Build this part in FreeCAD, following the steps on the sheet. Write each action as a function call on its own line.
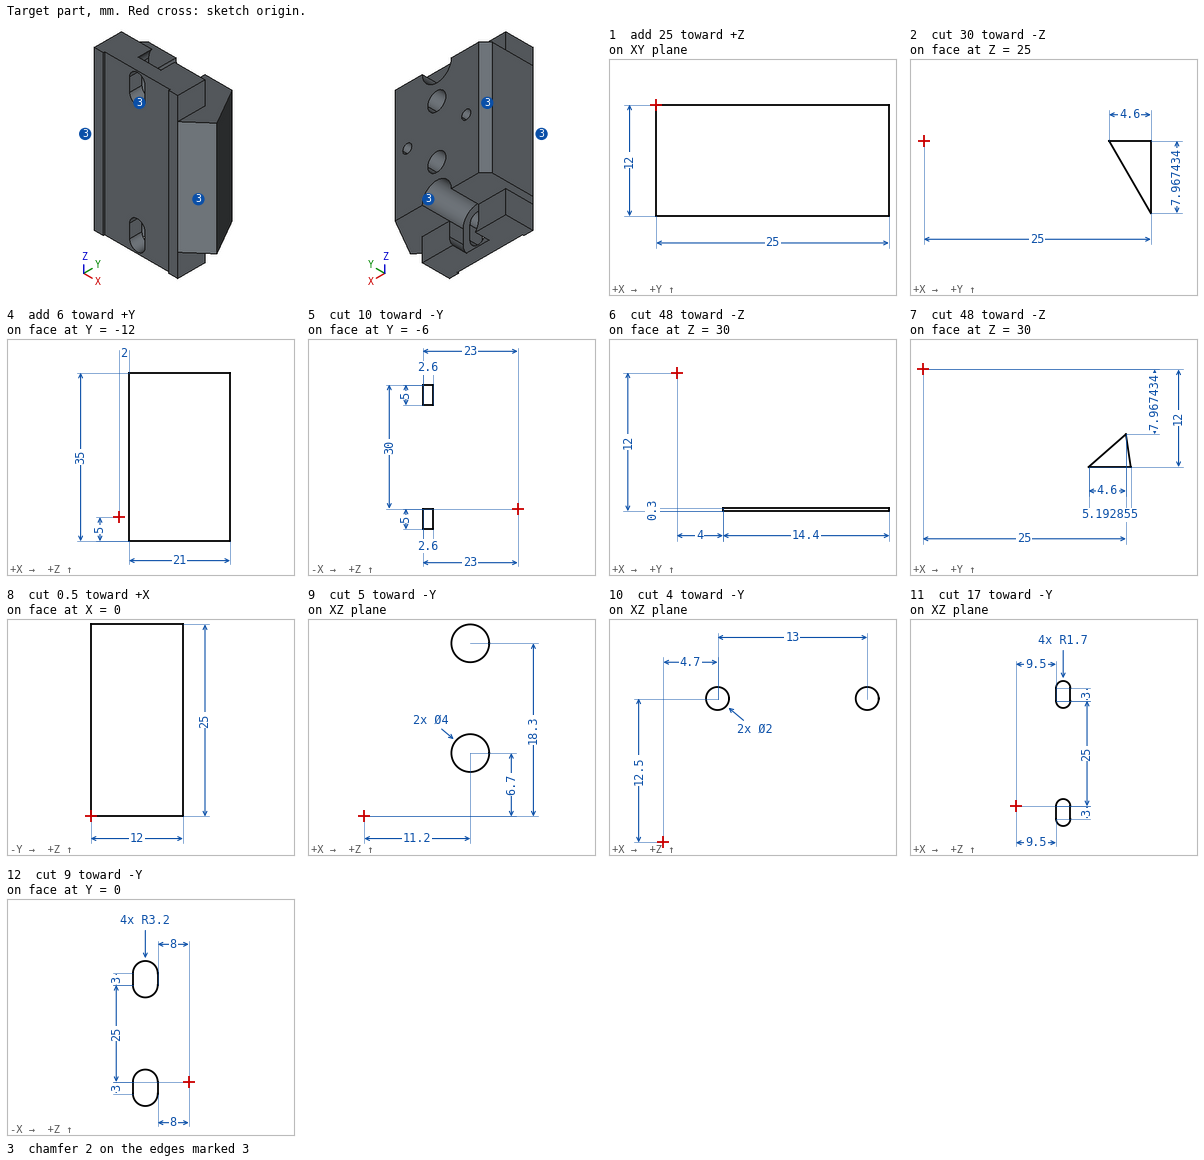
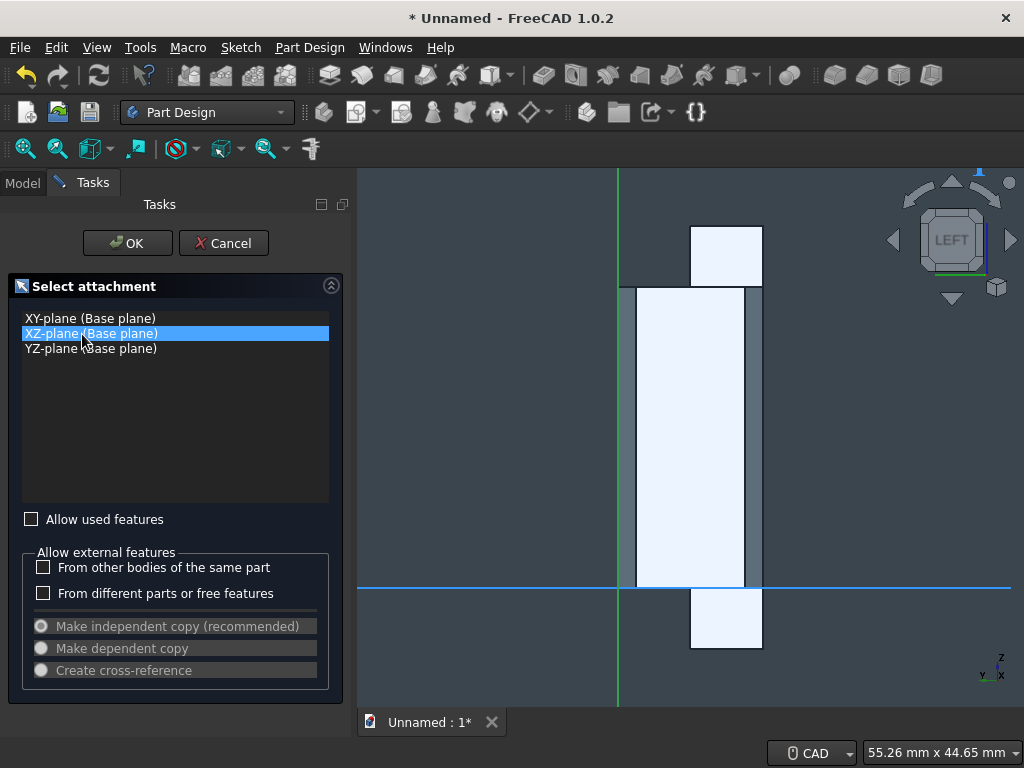
click(128, 243)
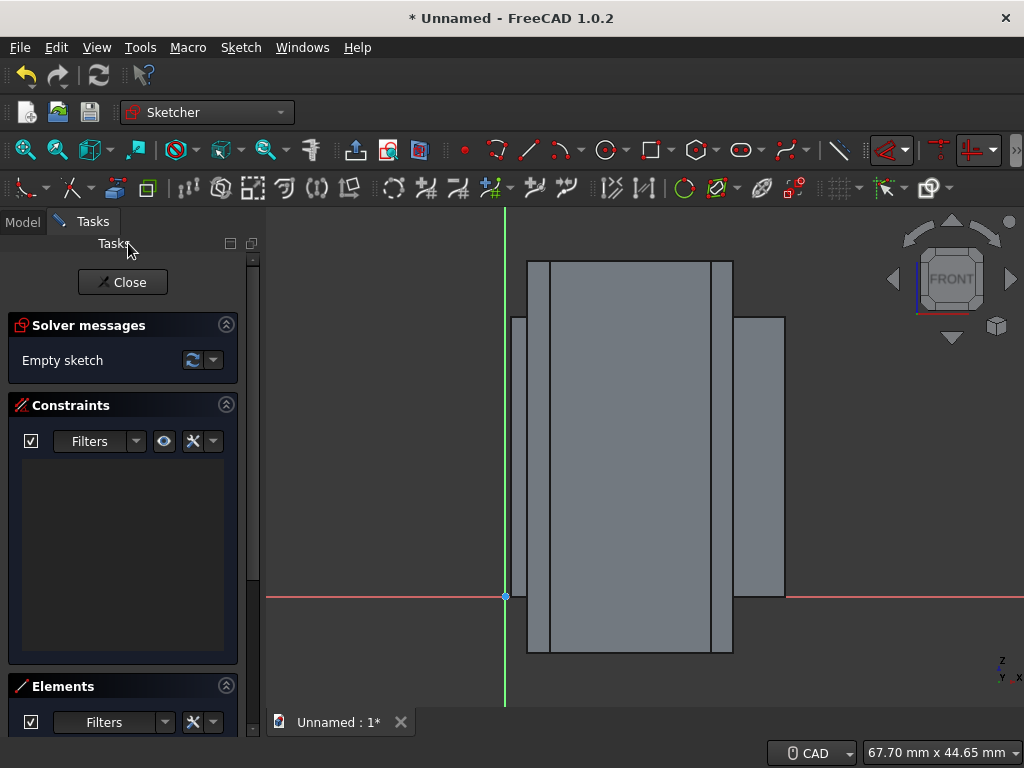
click(420, 150)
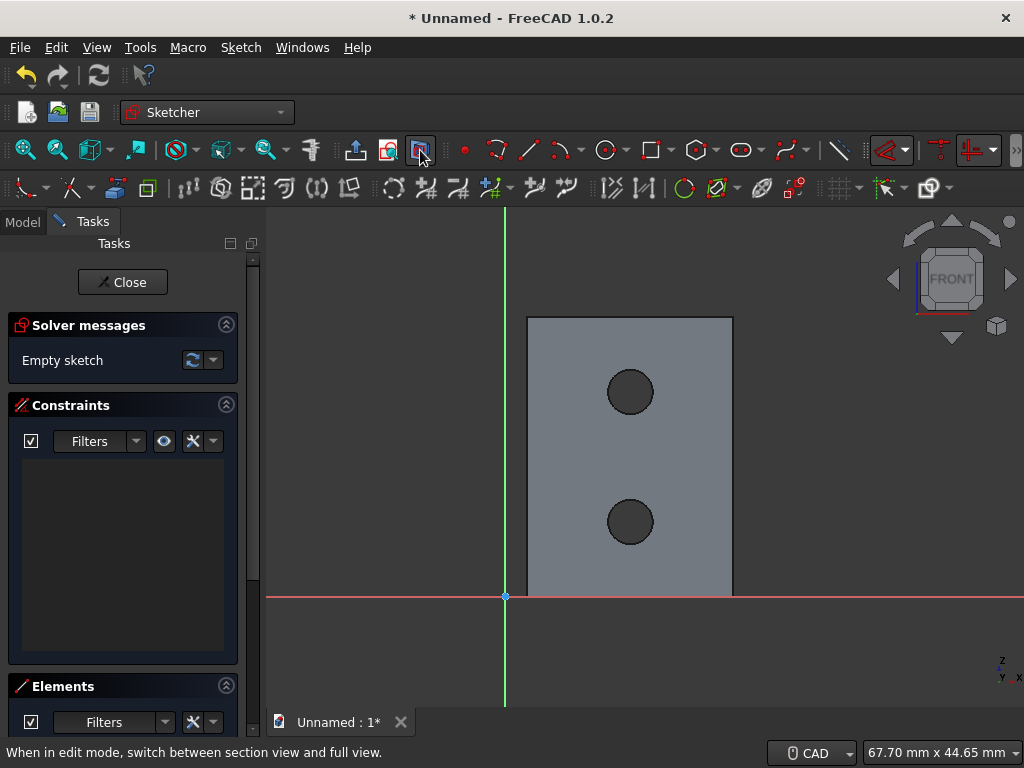
scroll(650, 600, up, 3)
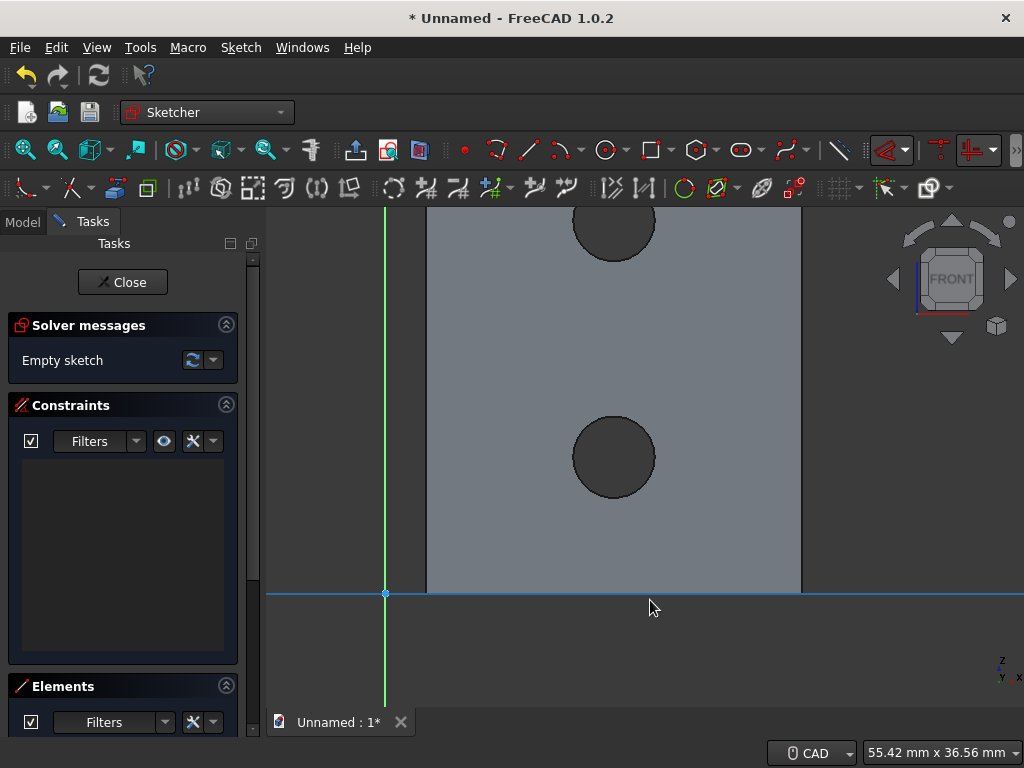
click(606, 150)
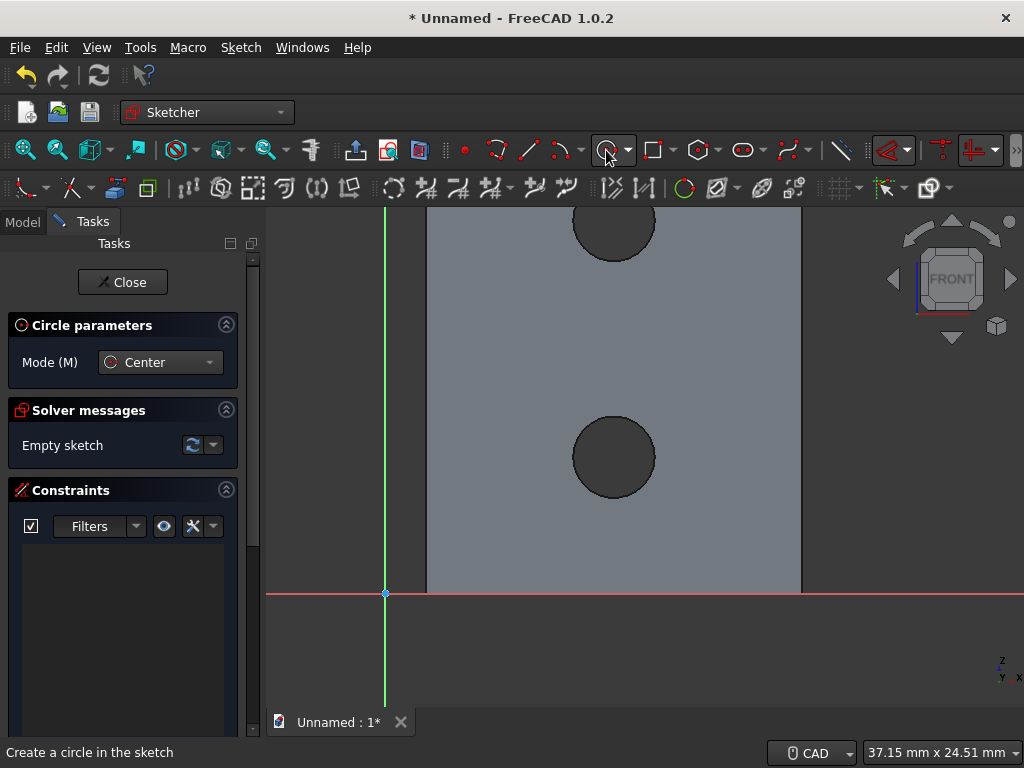
click(481, 339)
click(496, 324)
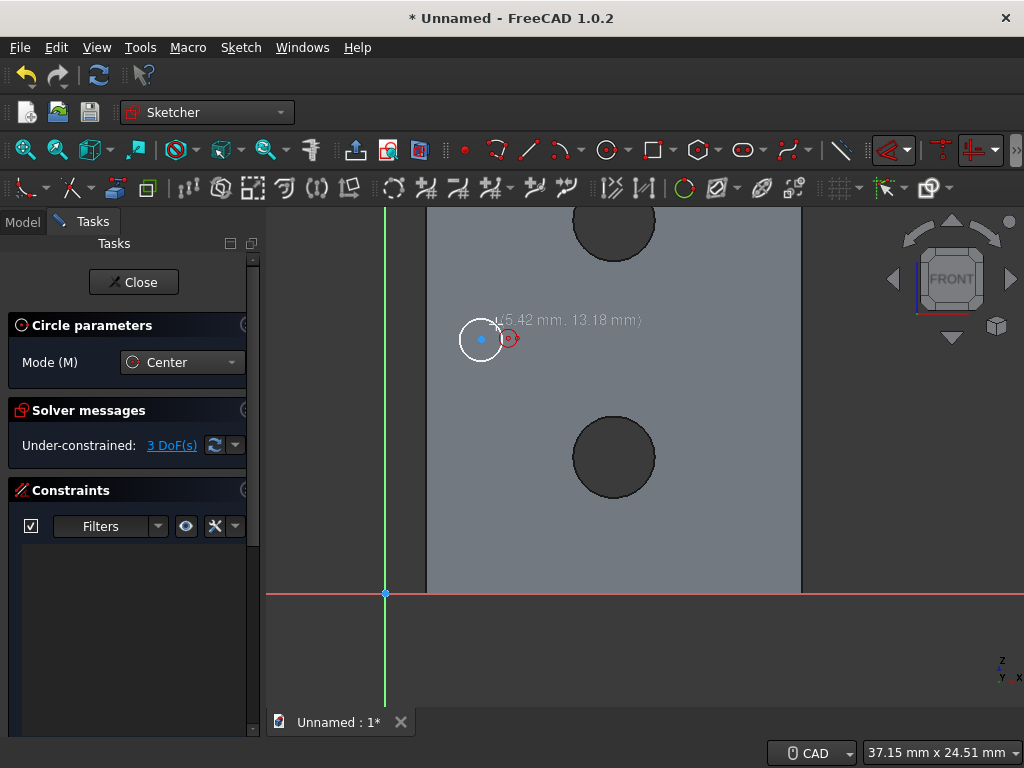
click(747, 339)
click(761, 324)
key(Escape)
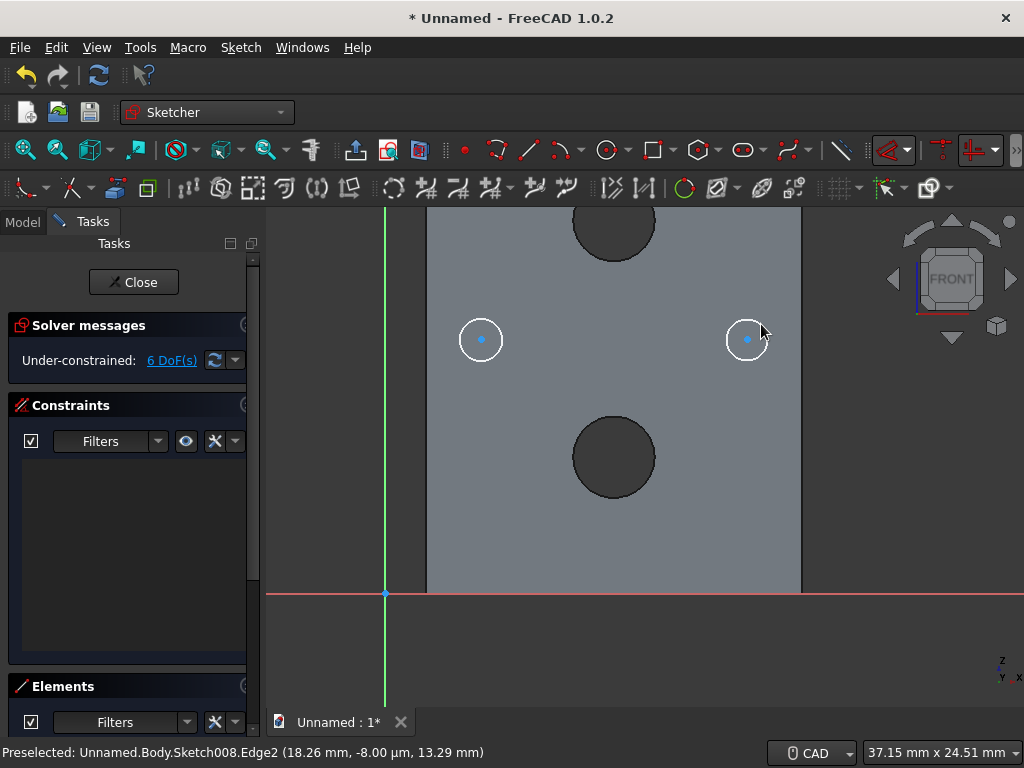
click(496, 325)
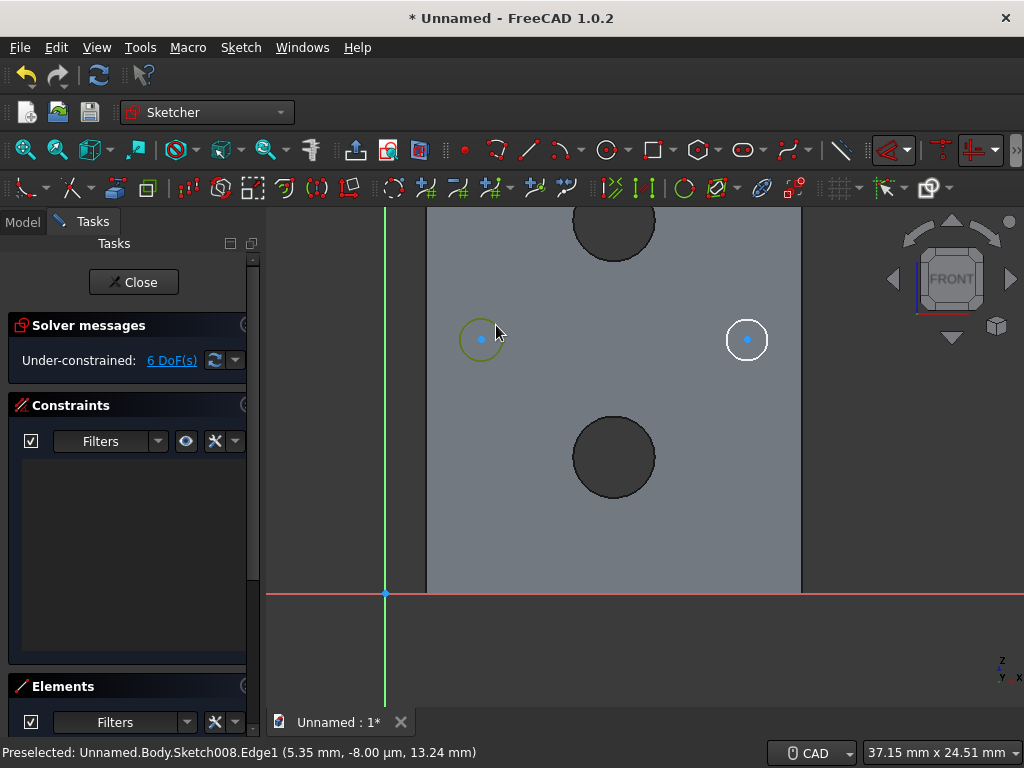
click(761, 325)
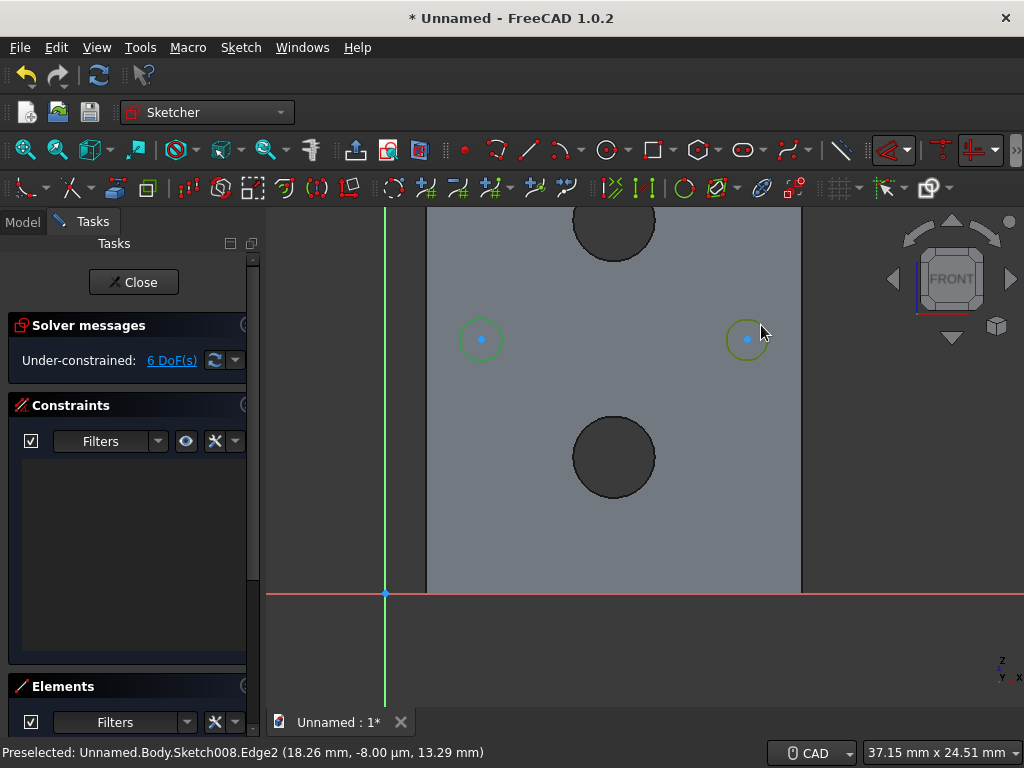
key(e)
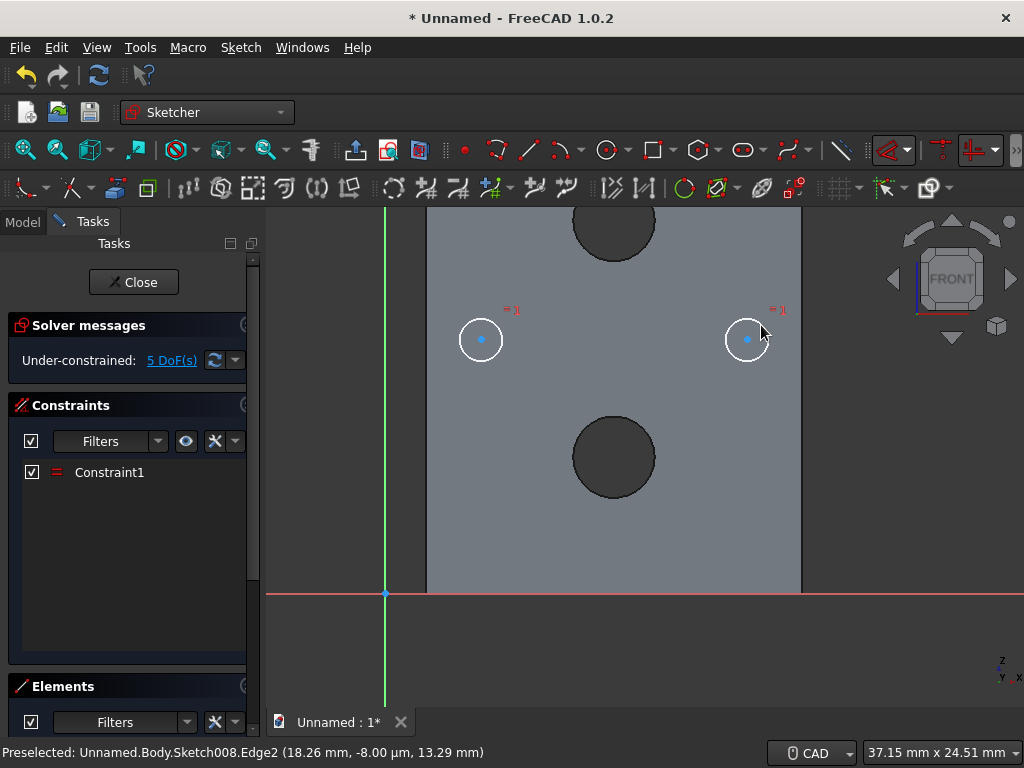
click(481, 340)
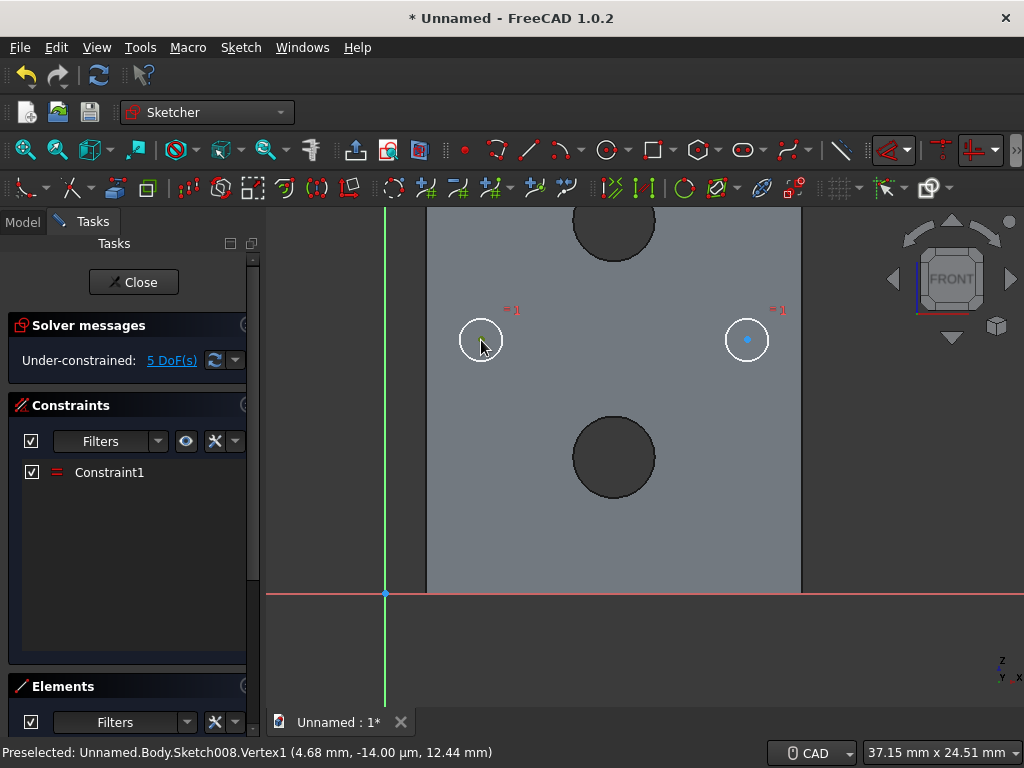
click(747, 340)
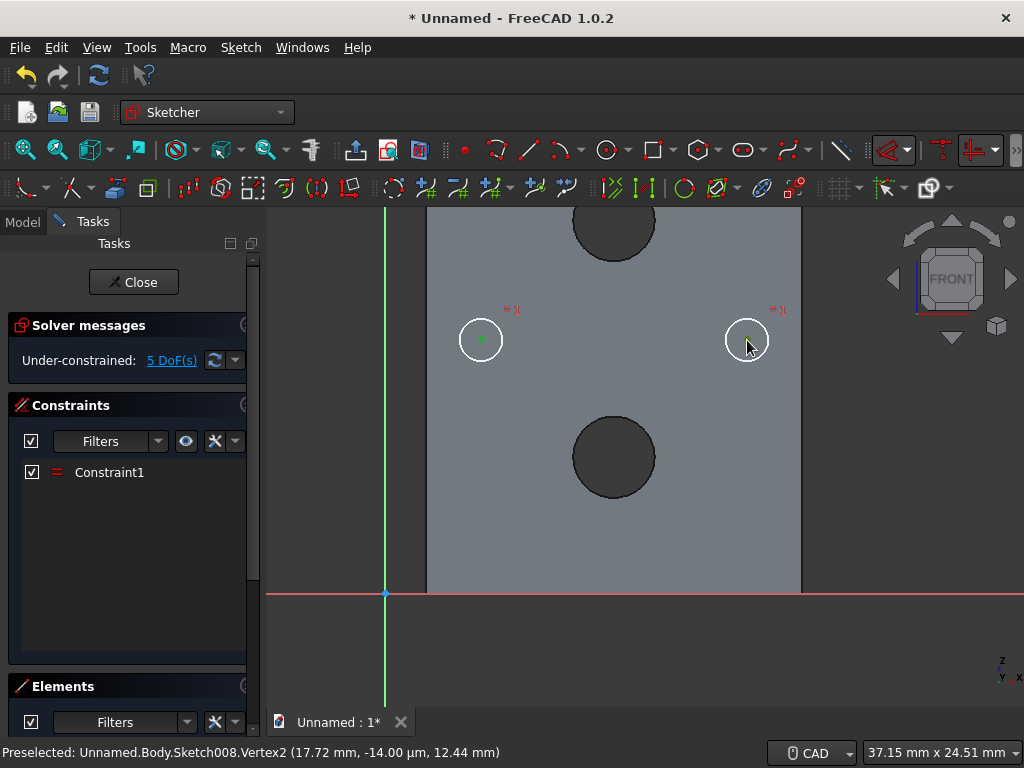
click(998, 150)